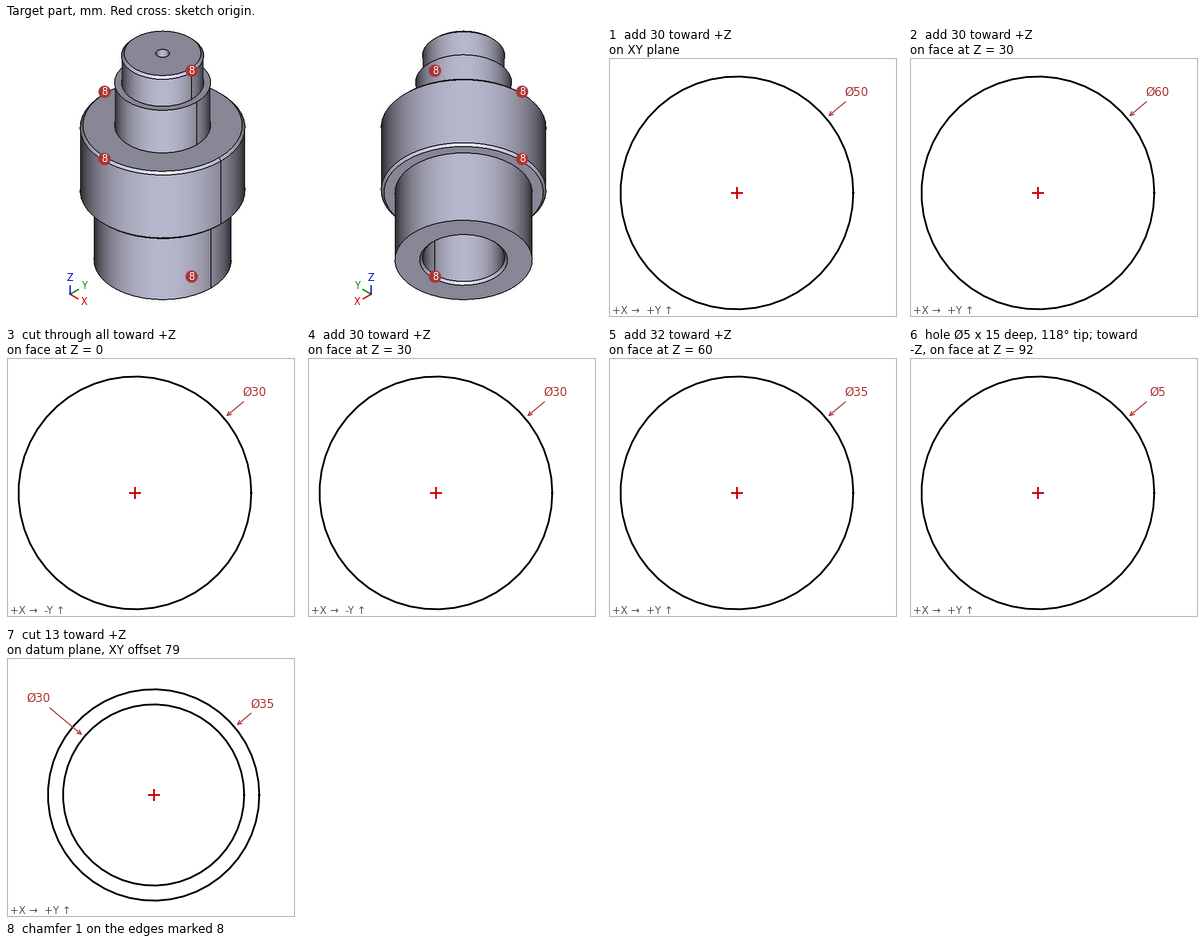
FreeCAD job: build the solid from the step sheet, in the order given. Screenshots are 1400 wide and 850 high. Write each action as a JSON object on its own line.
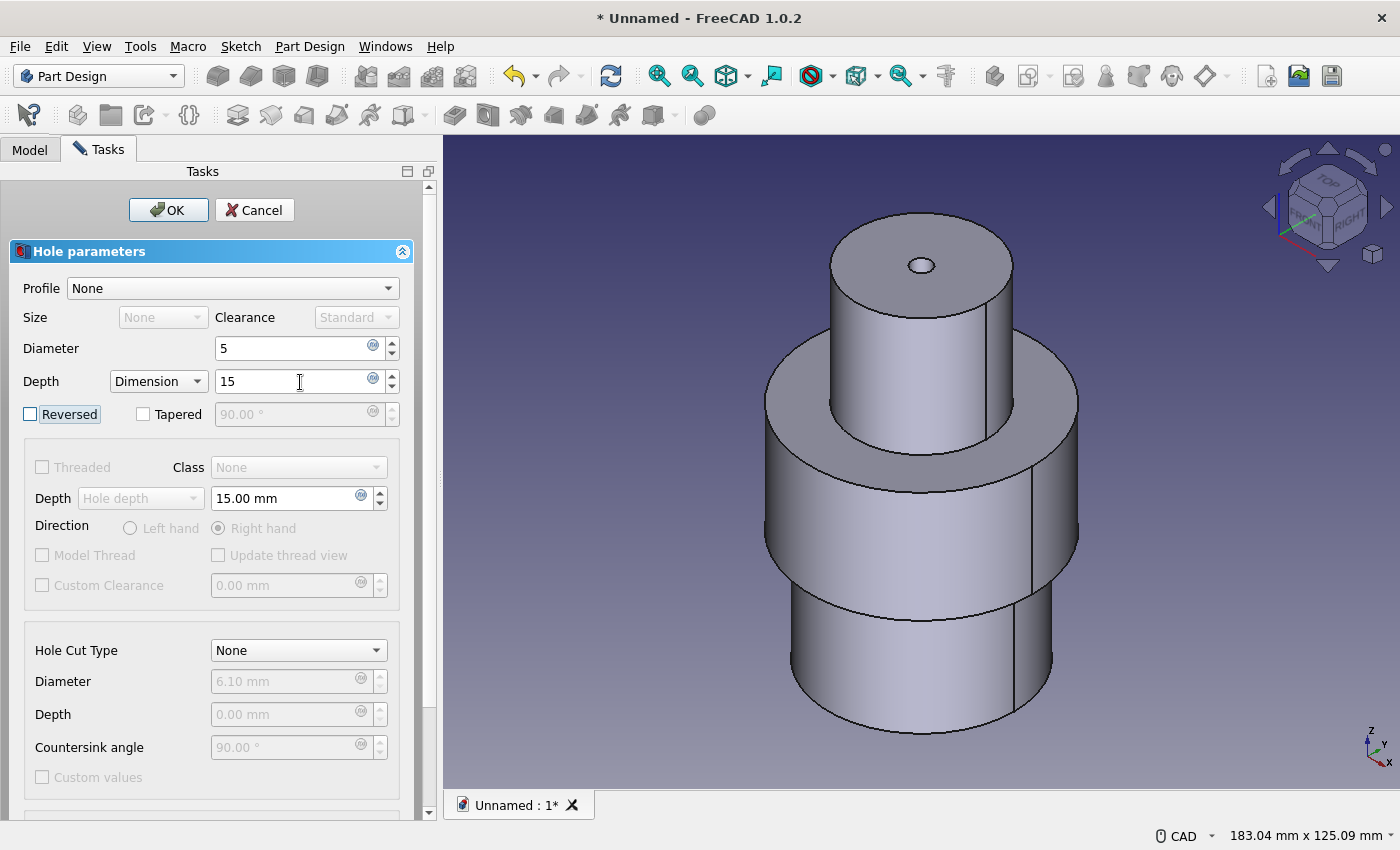
{"action": "left_click", "coordinate": [169, 210]}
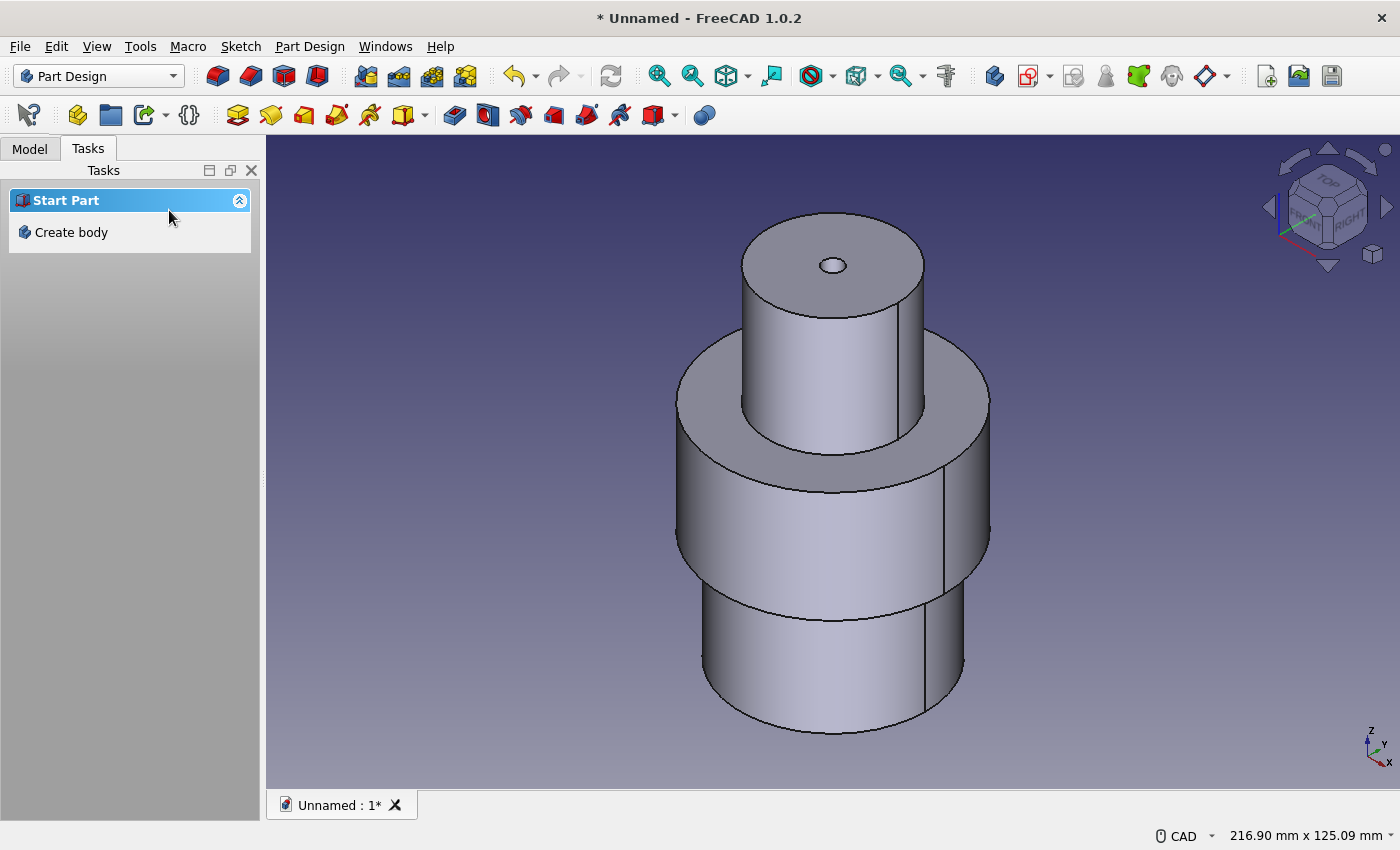
{"action": "left_click", "coordinate": [30, 148]}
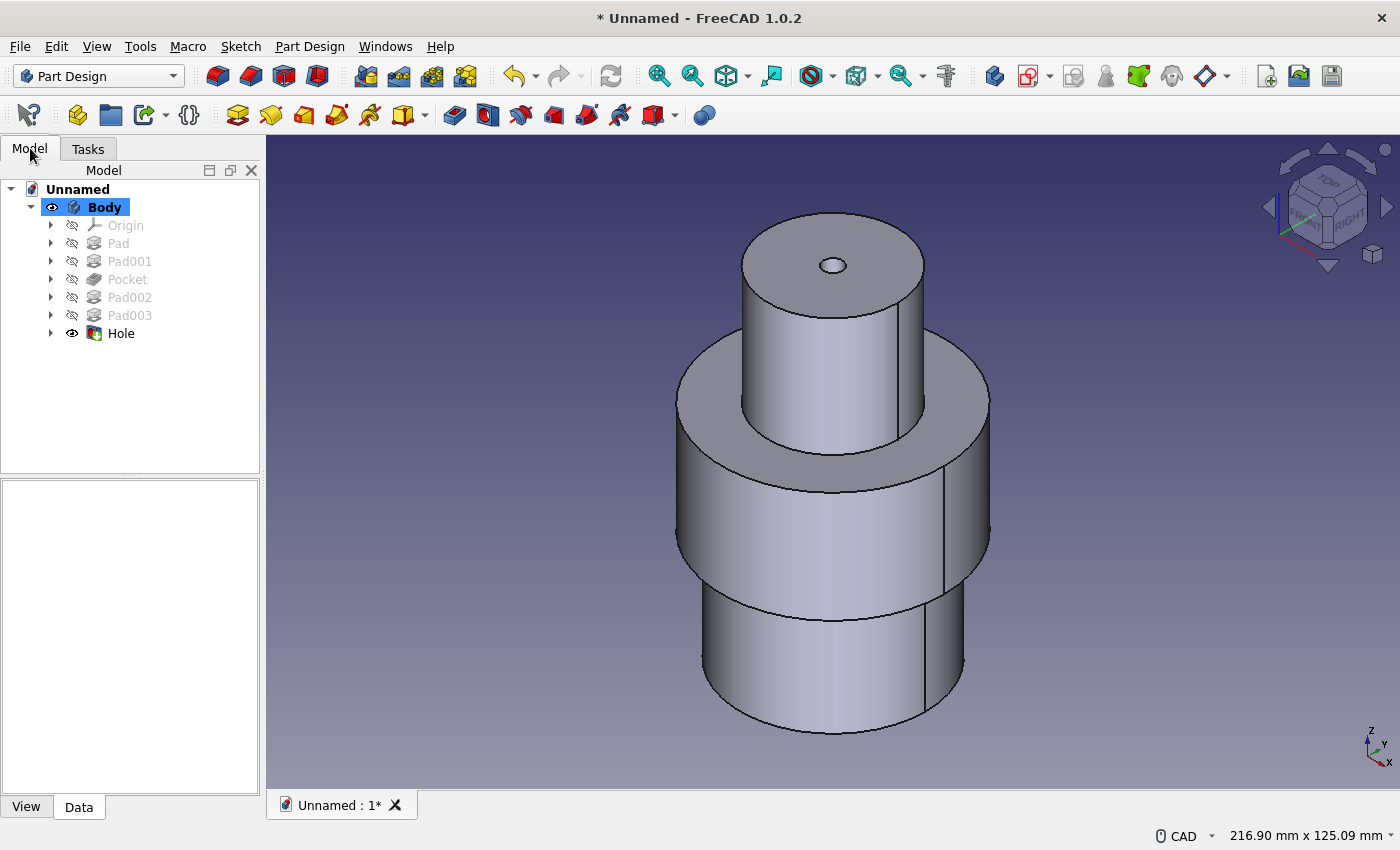
{"action": "left_click", "coordinate": [51, 225]}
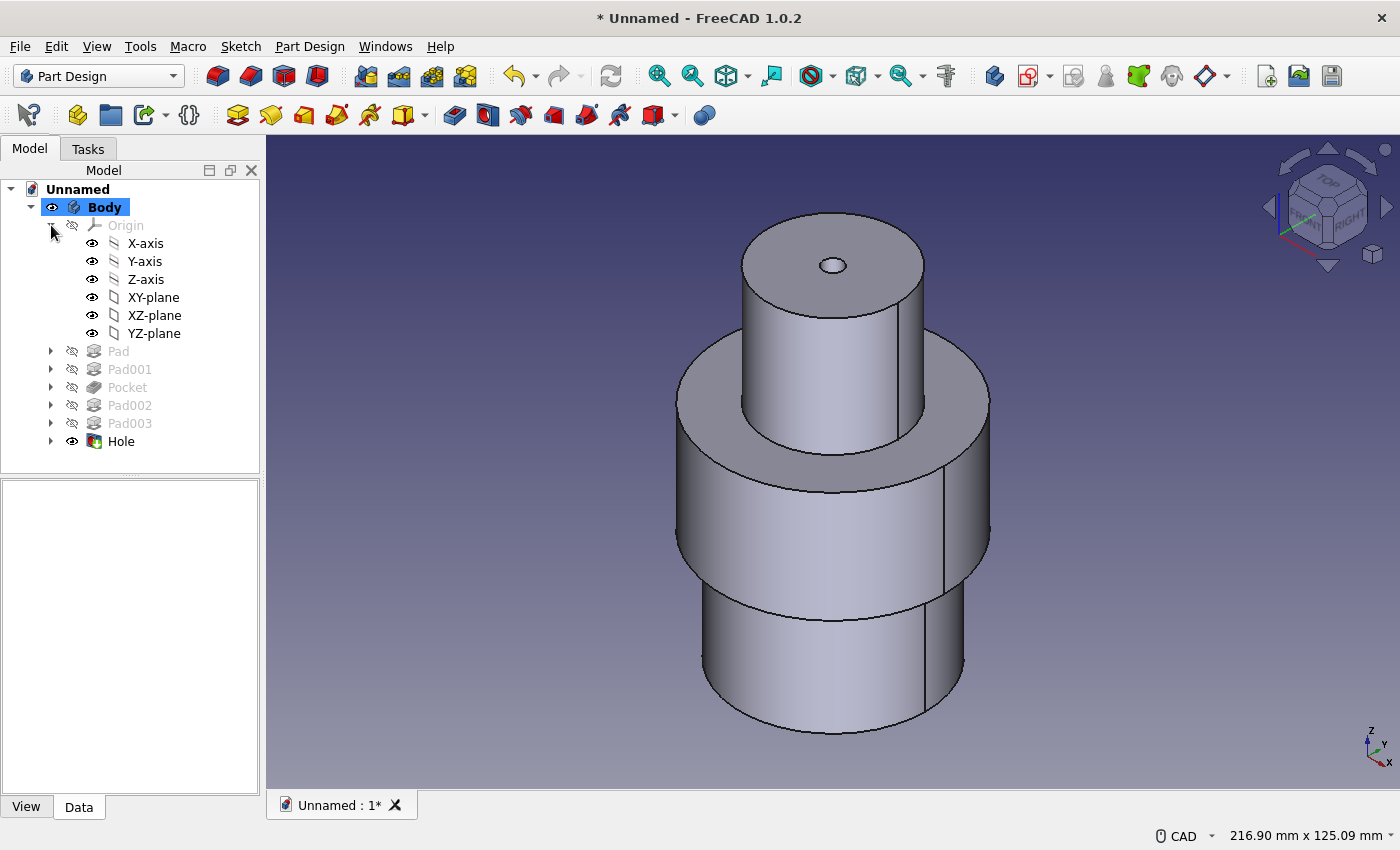
{"action": "left_click", "coordinate": [137, 297]}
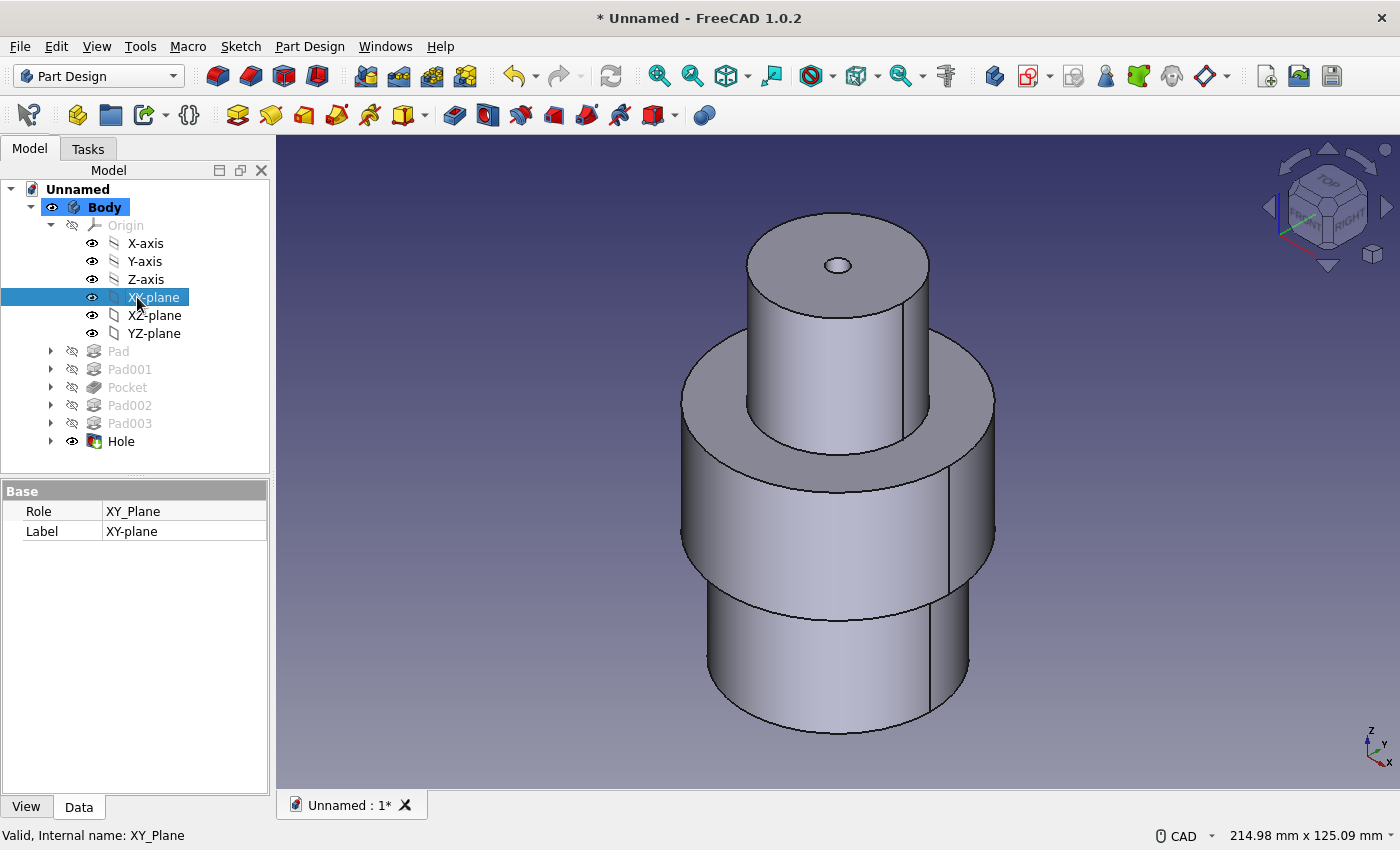
{"action": "left_click", "coordinate": [1204, 76]}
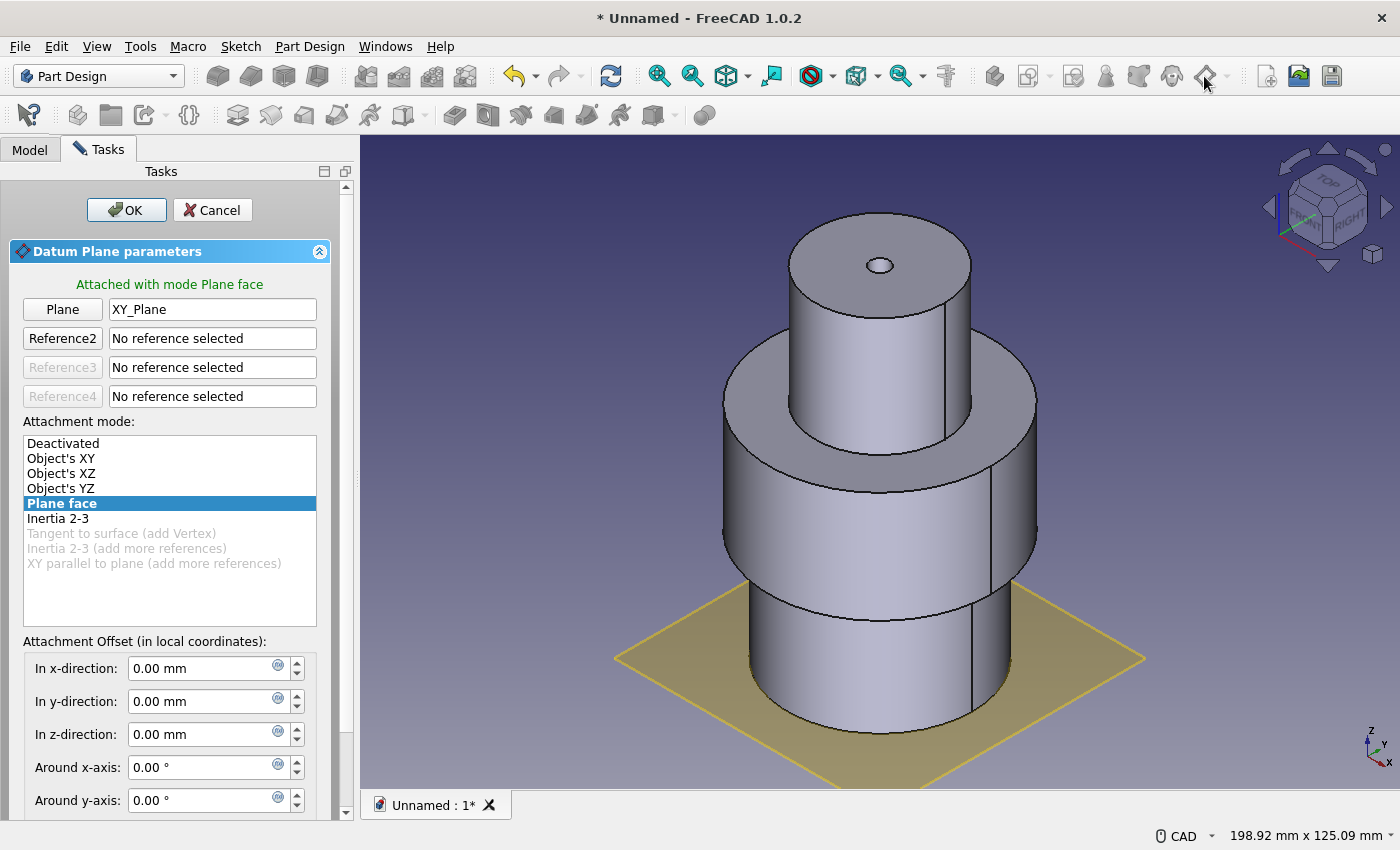
{"action": "triple_click", "coordinate": [210, 734]}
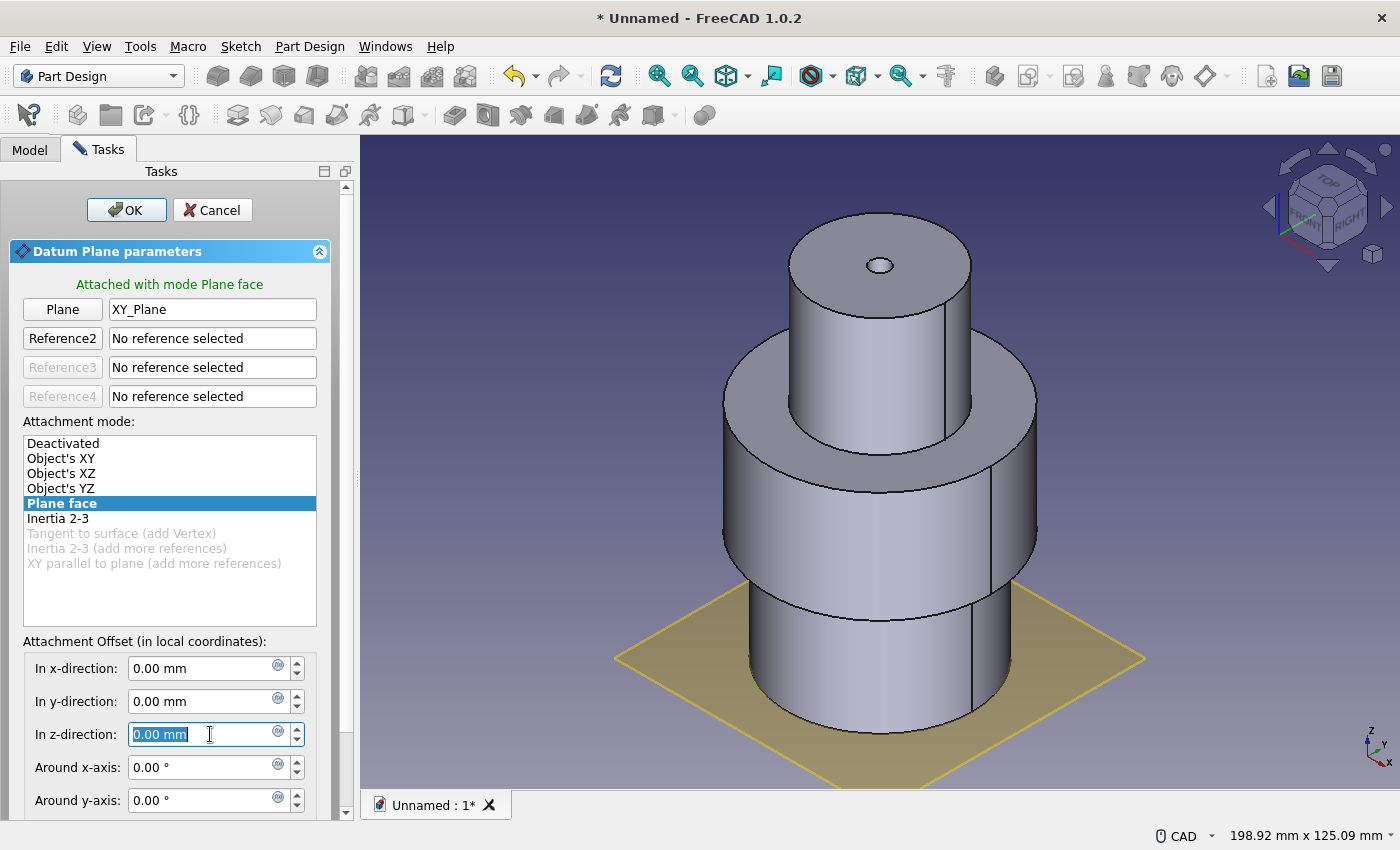
{"action": "type", "text": "79"}
{"action": "key", "text": "Tab"}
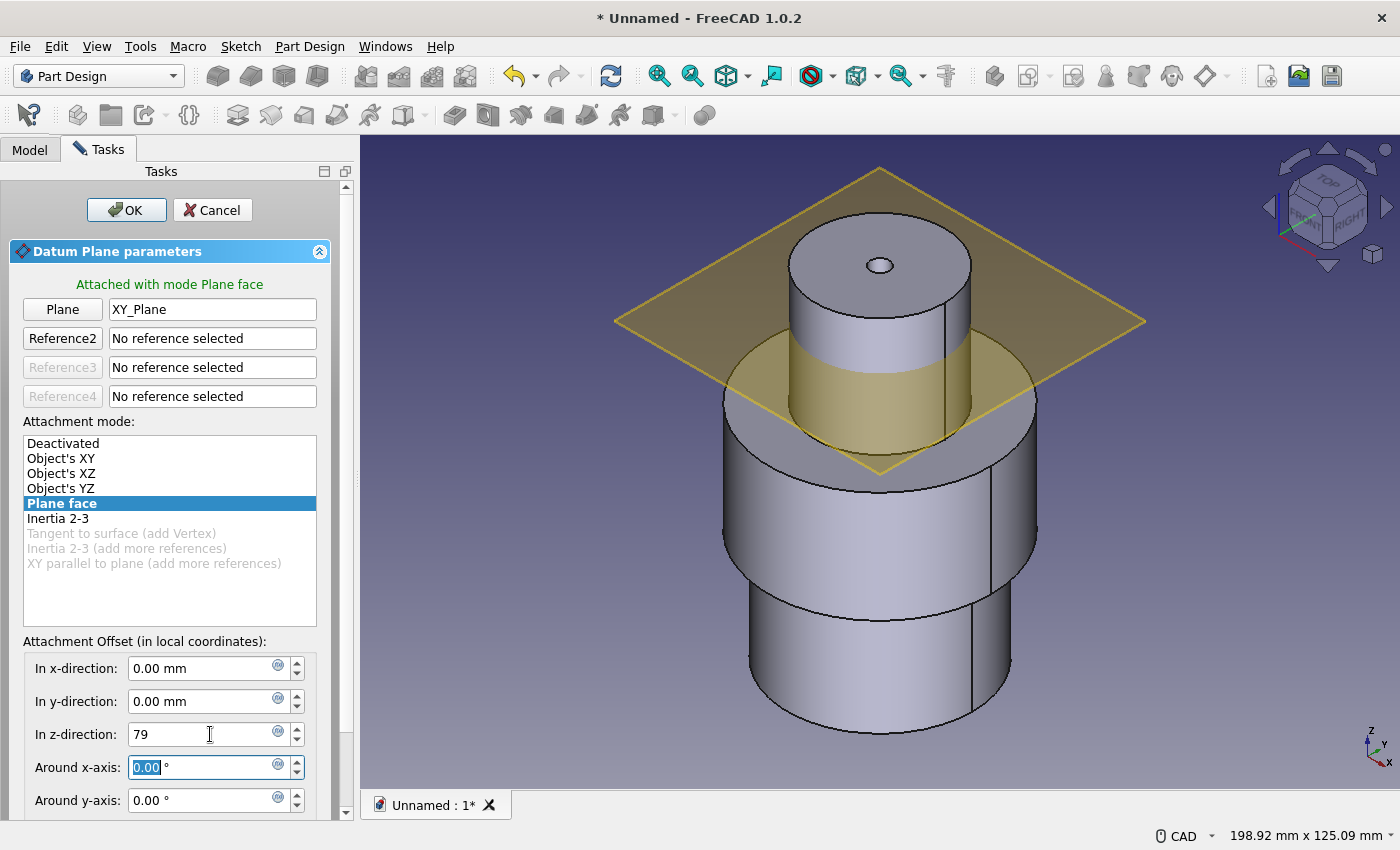
{"action": "left_click", "coordinate": [127, 210]}